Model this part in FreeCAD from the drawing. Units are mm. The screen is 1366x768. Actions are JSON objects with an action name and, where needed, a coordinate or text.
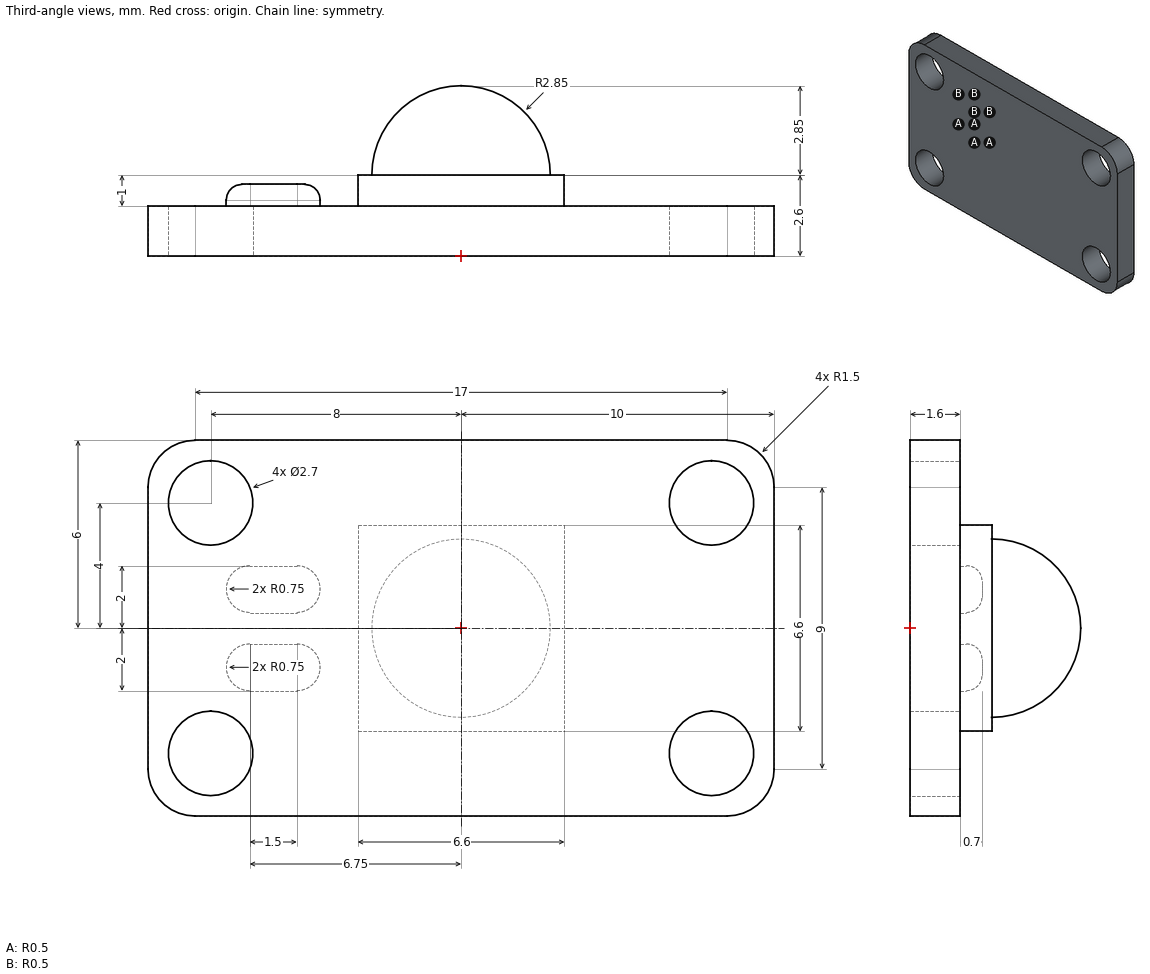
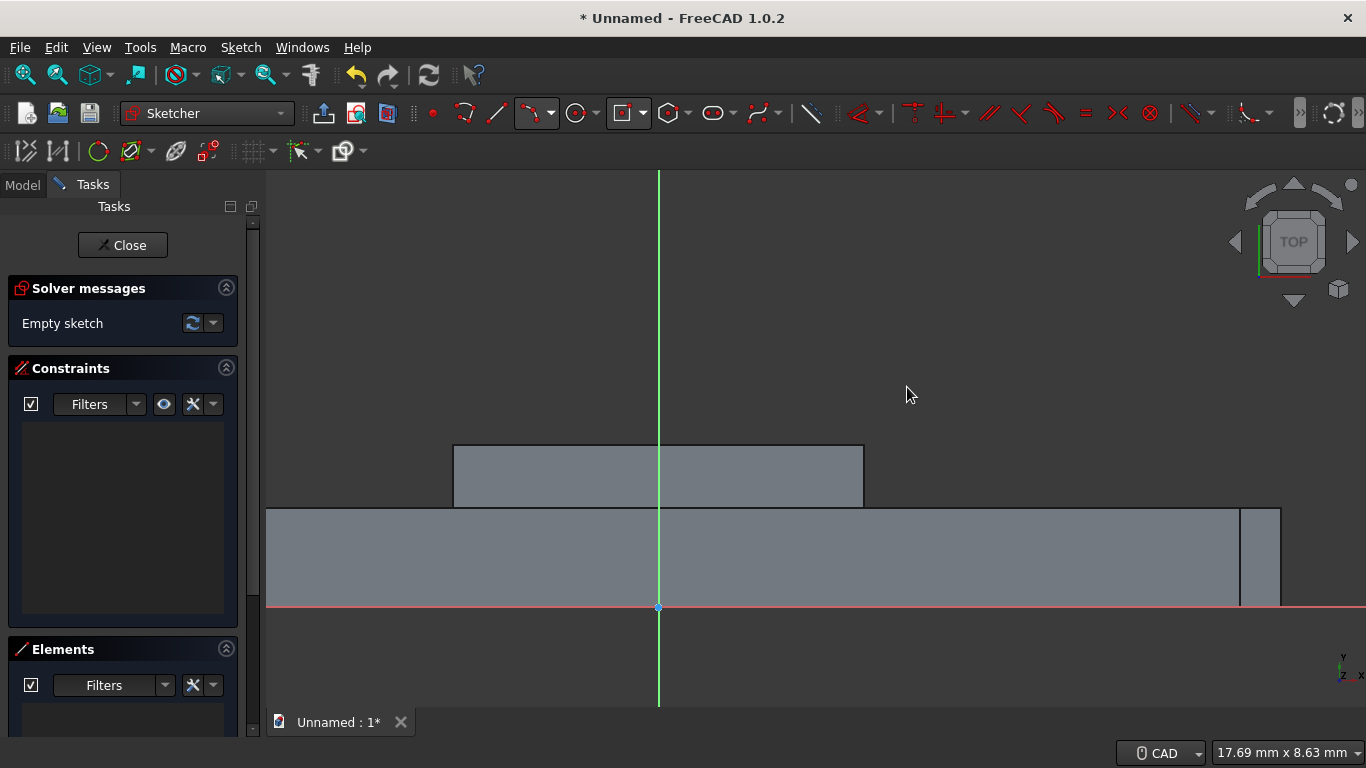
{"action": "key", "text": "g m"}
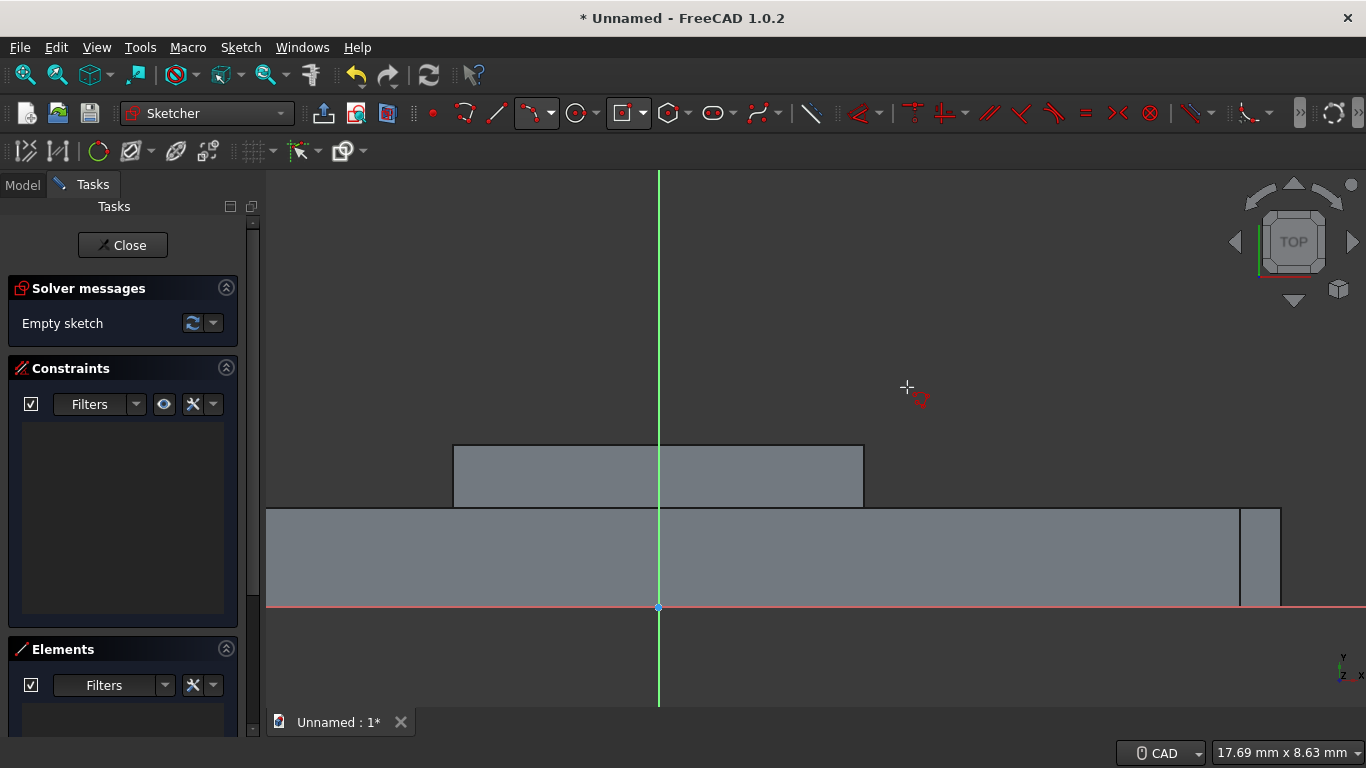
{"action": "left_click", "coordinate": [659, 268]}
{"action": "left_click", "coordinate": [668, 445]}
{"action": "left_click", "coordinate": [836, 445]}
{"action": "right_click", "coordinate": [836, 445]}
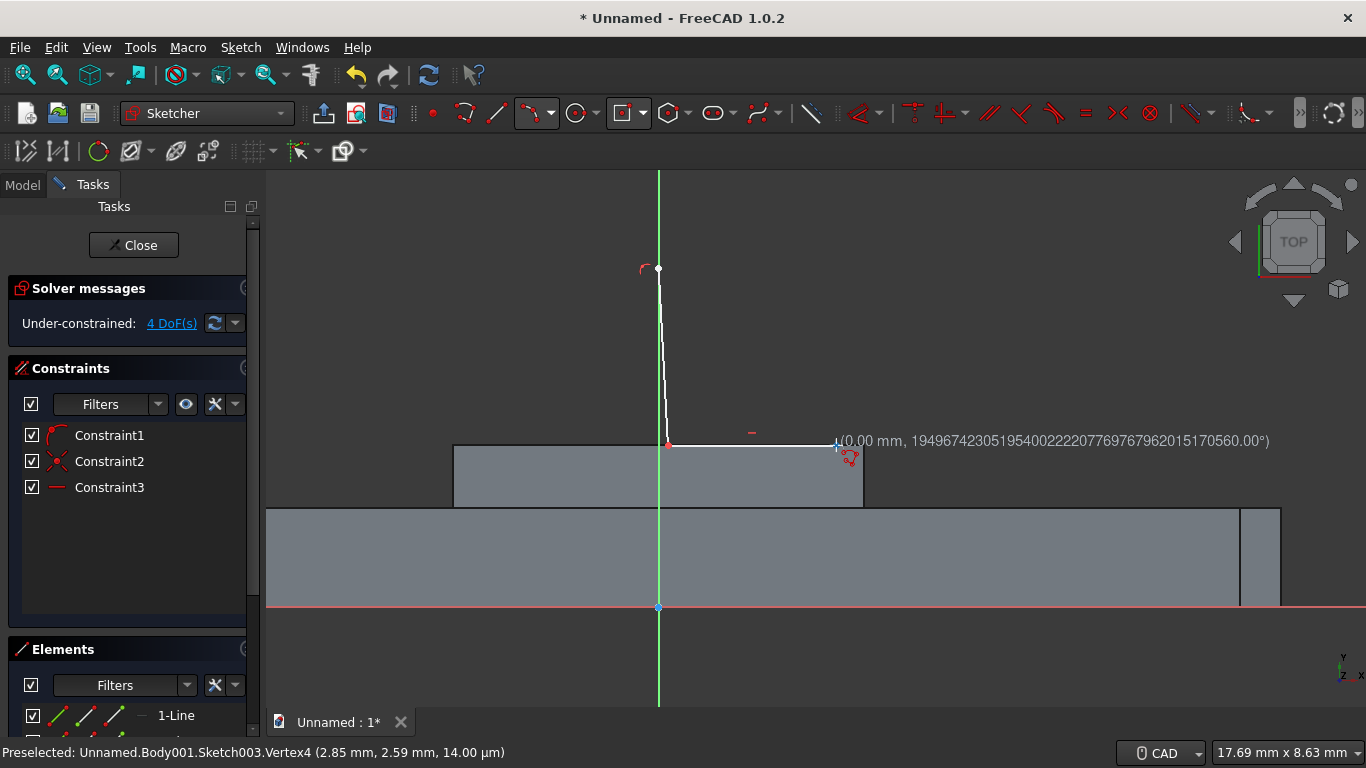
{"action": "key", "text": "g 3 a"}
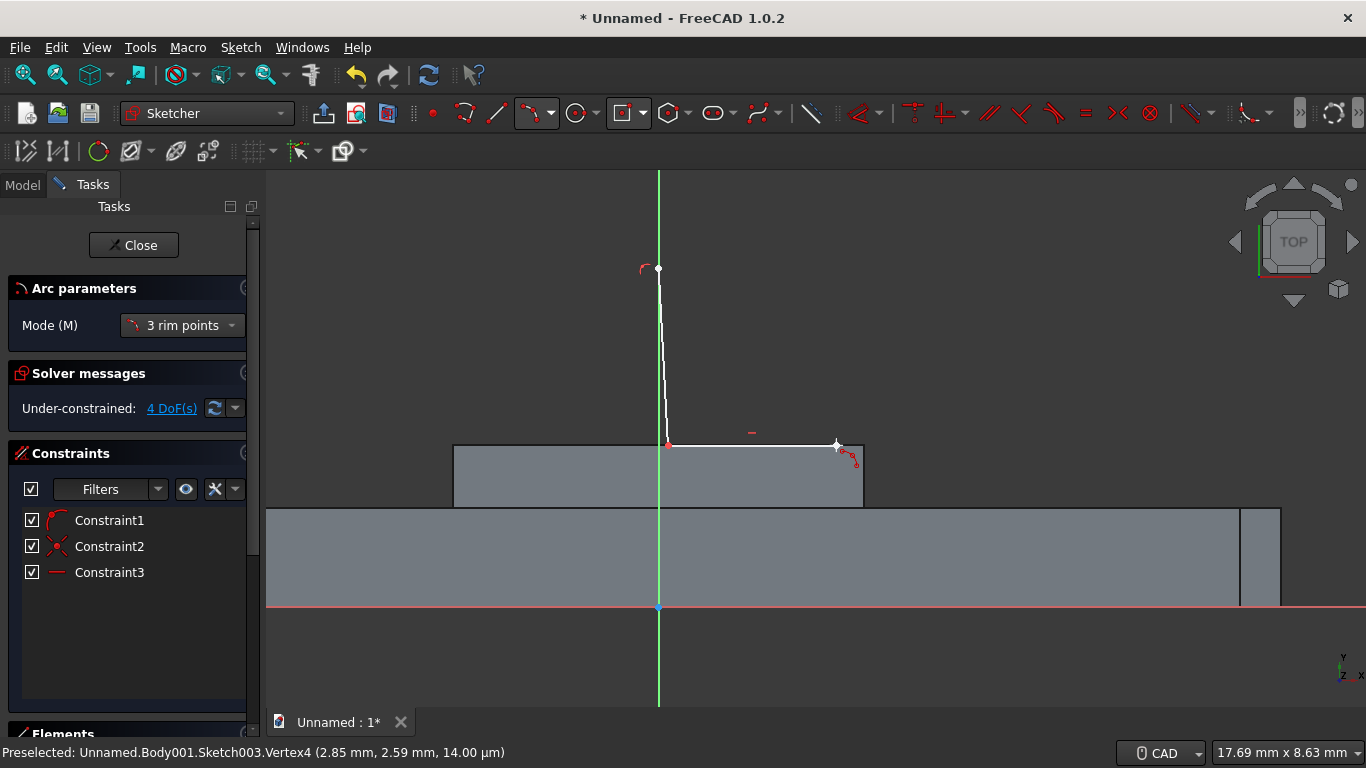
{"action": "left_click", "coordinate": [836, 446]}
{"action": "left_click", "coordinate": [659, 269]}
{"action": "left_click", "coordinate": [784, 320]}
{"action": "key", "text": "Escape"}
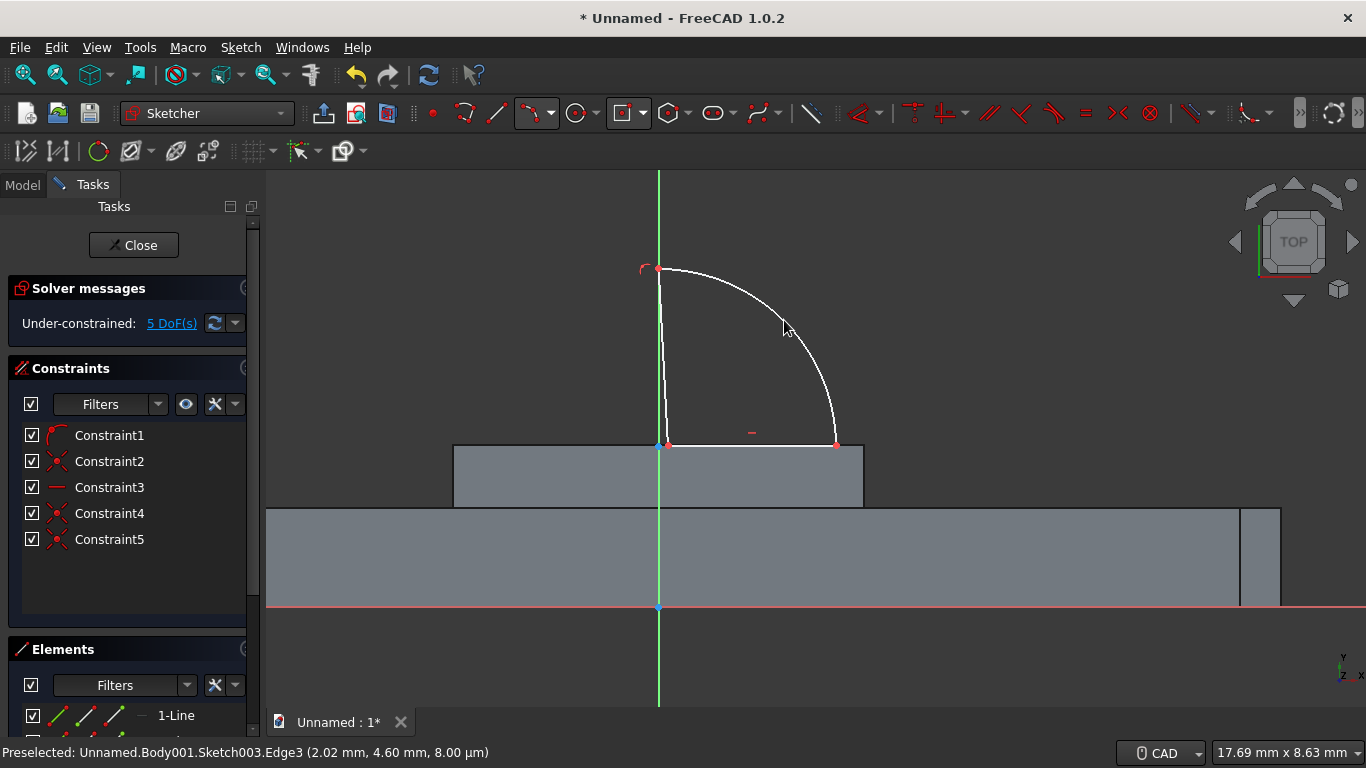
{"action": "left_click", "coordinate": [661, 322]}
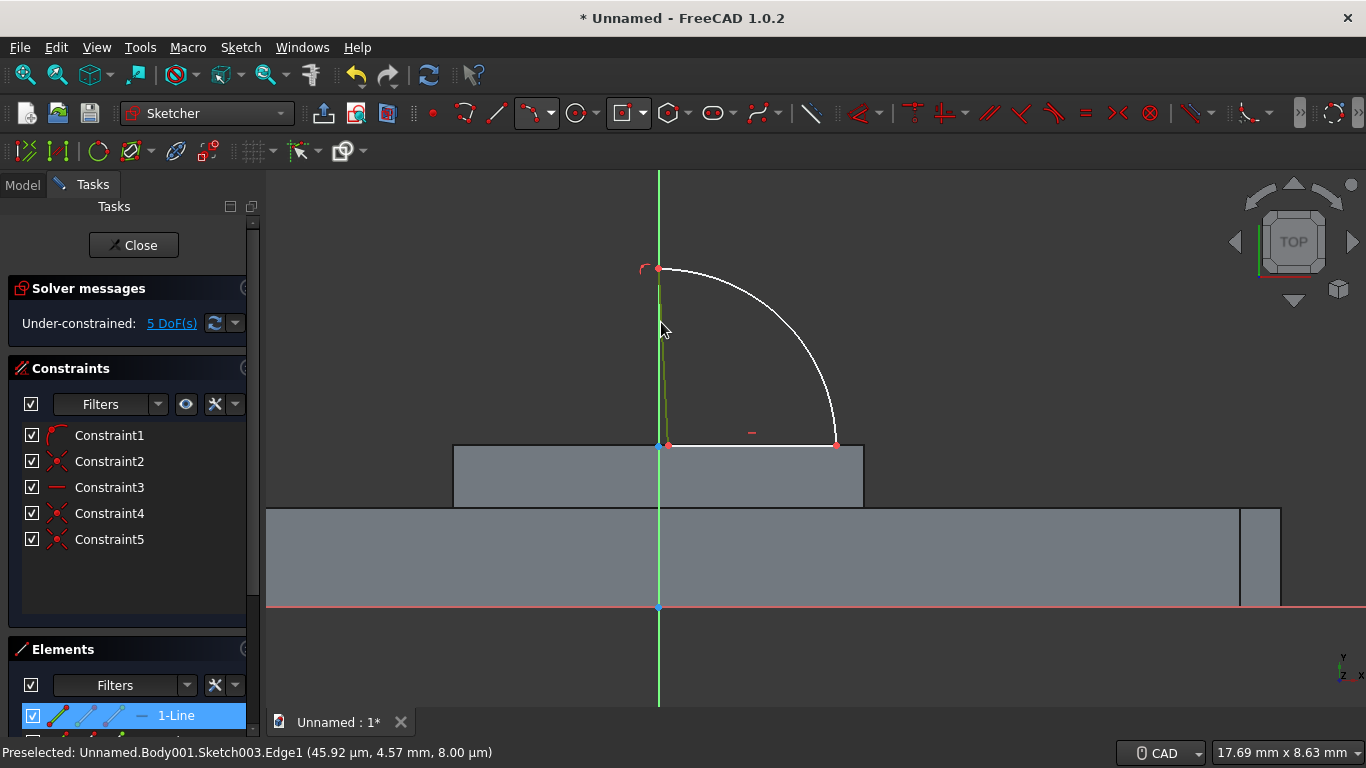
{"action": "left_click", "coordinate": [968, 114]}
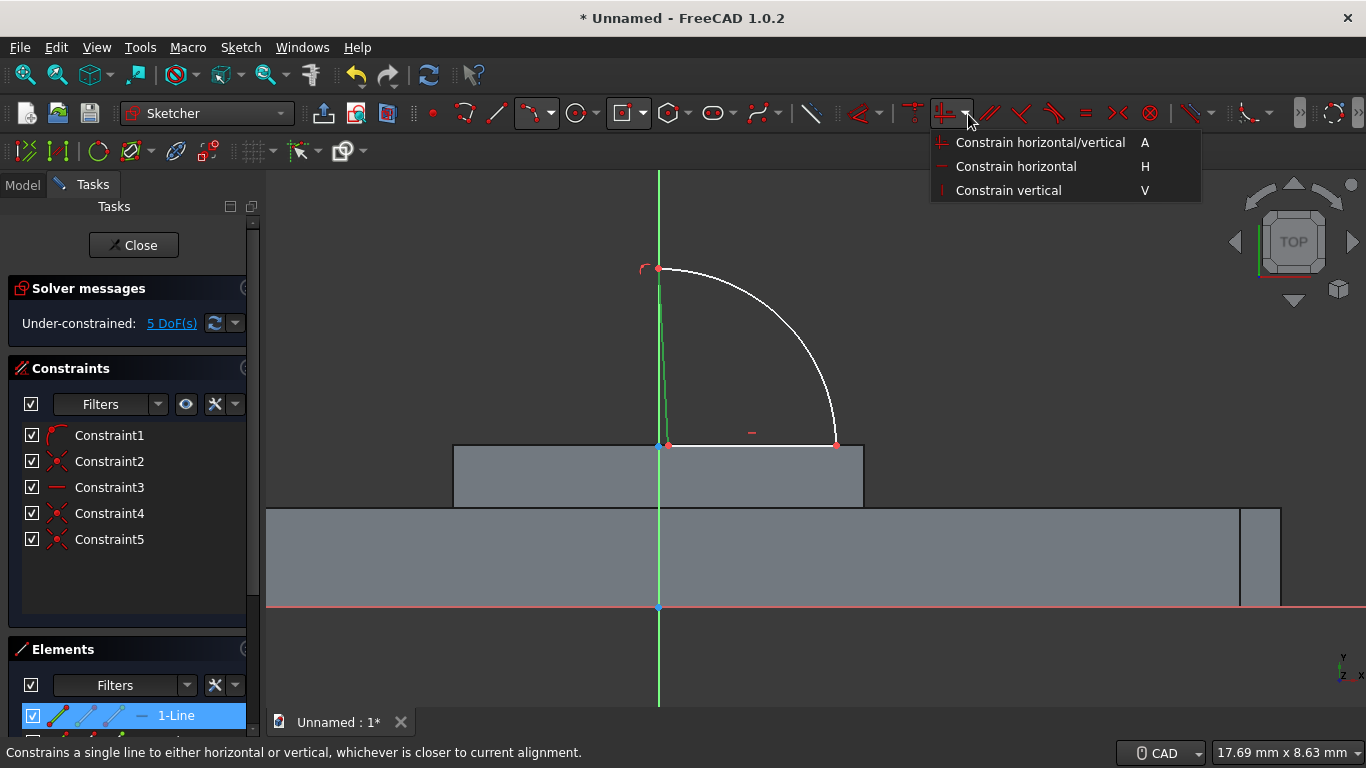
{"action": "left_click", "coordinate": [1066, 190]}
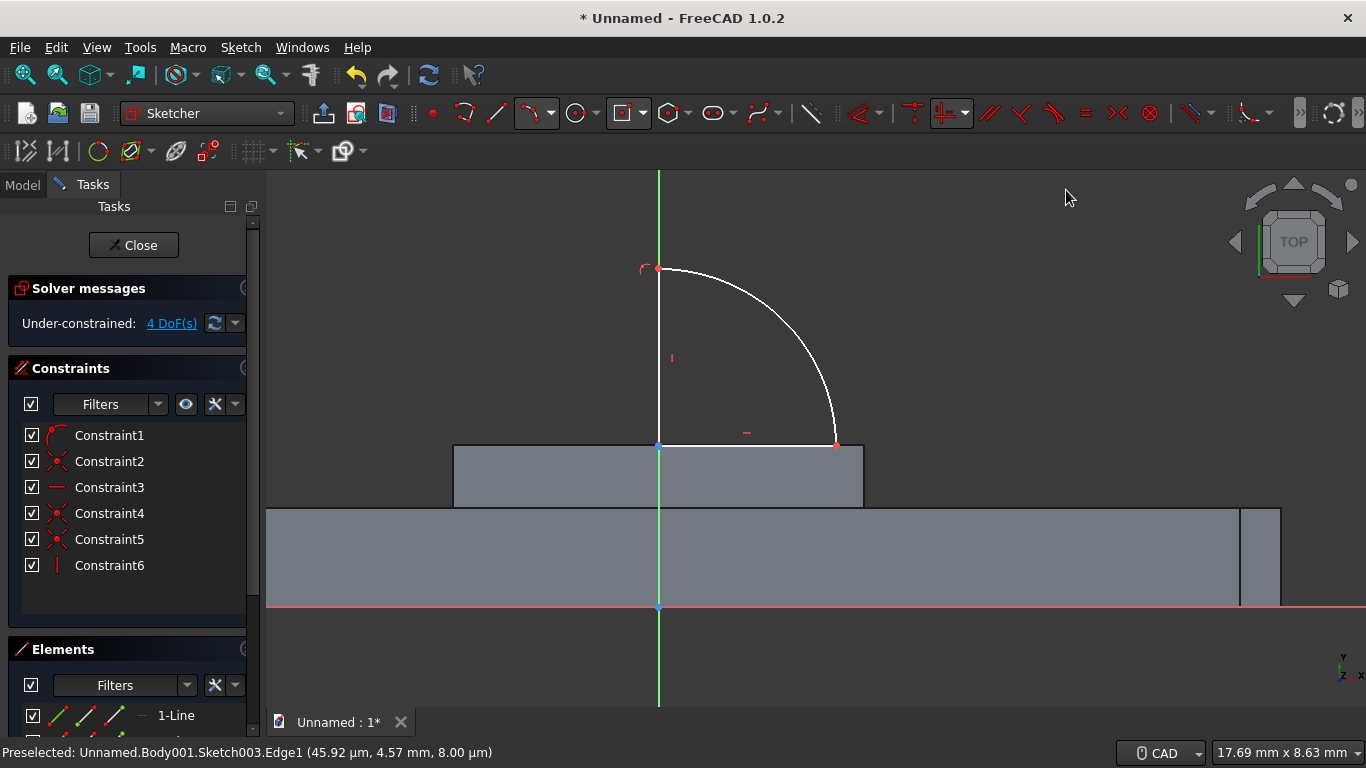
{"action": "left_click", "coordinate": [658, 447]}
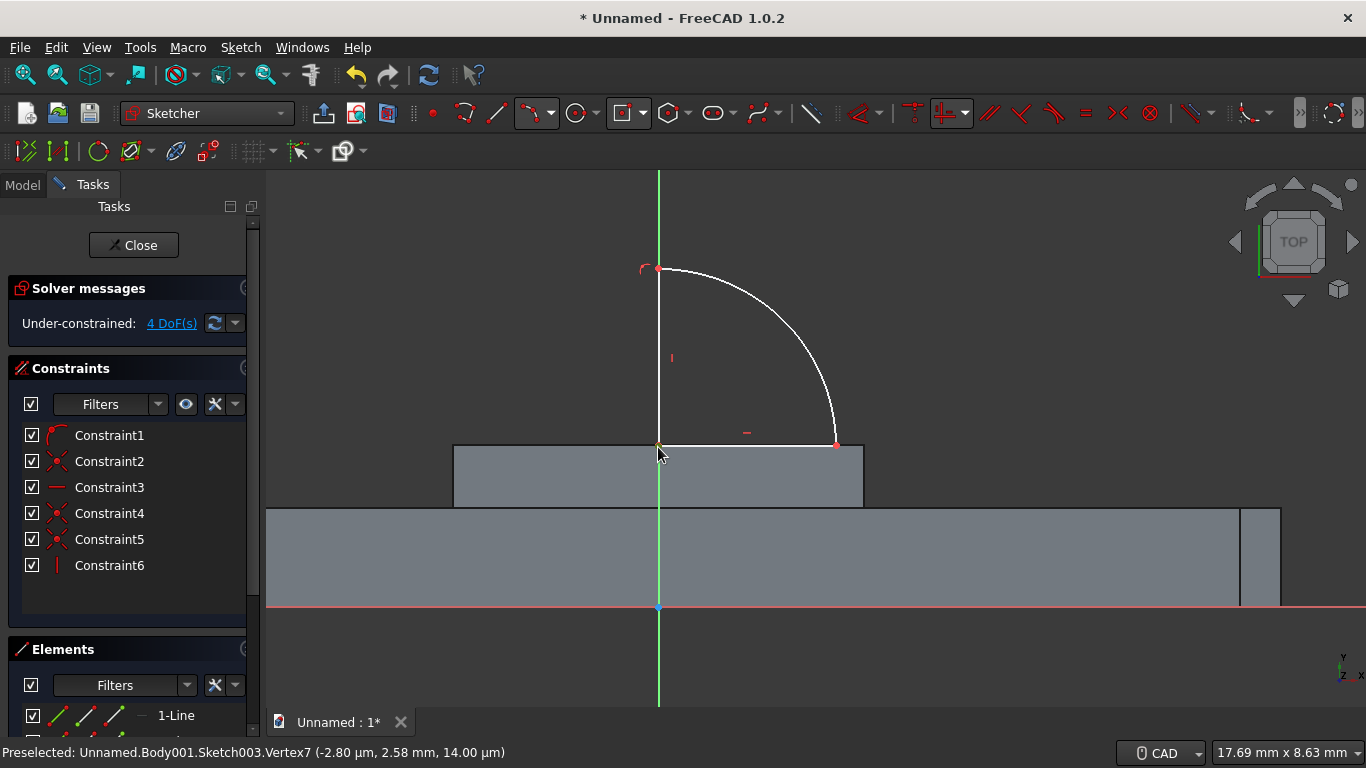
{"action": "left_click", "coordinate": [659, 645]}